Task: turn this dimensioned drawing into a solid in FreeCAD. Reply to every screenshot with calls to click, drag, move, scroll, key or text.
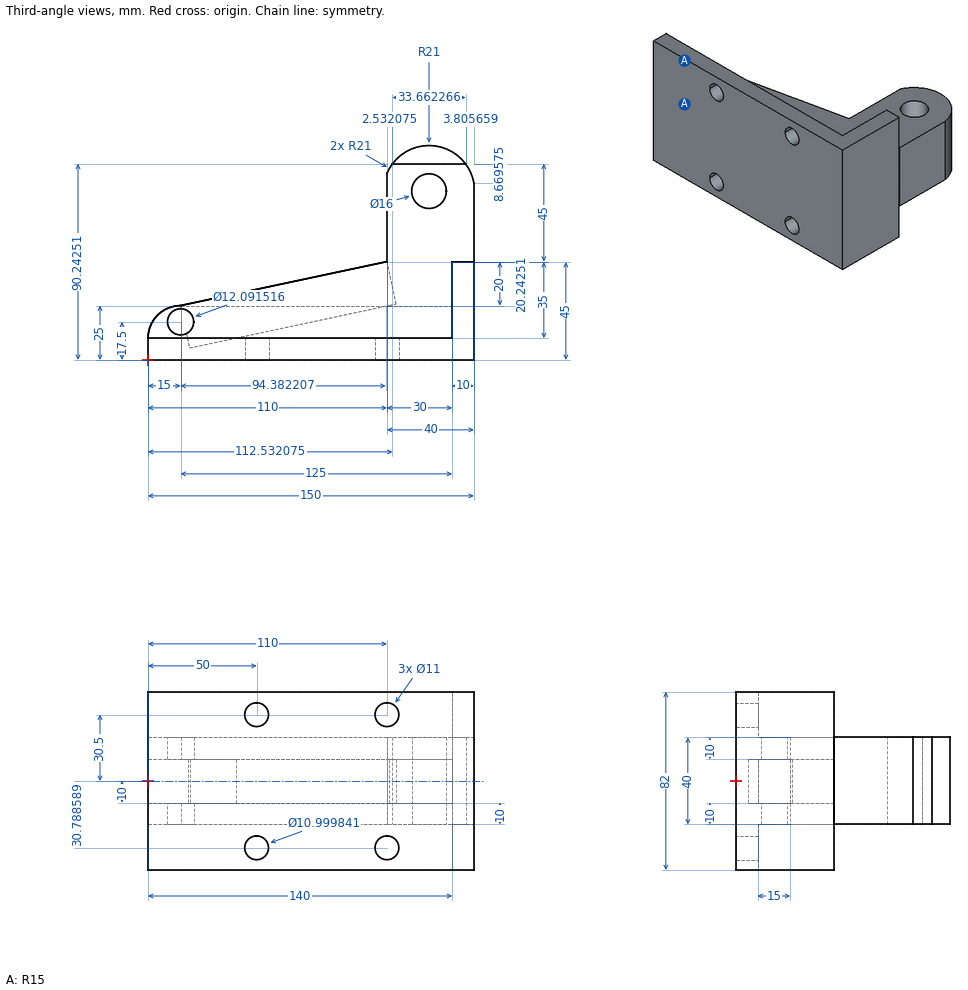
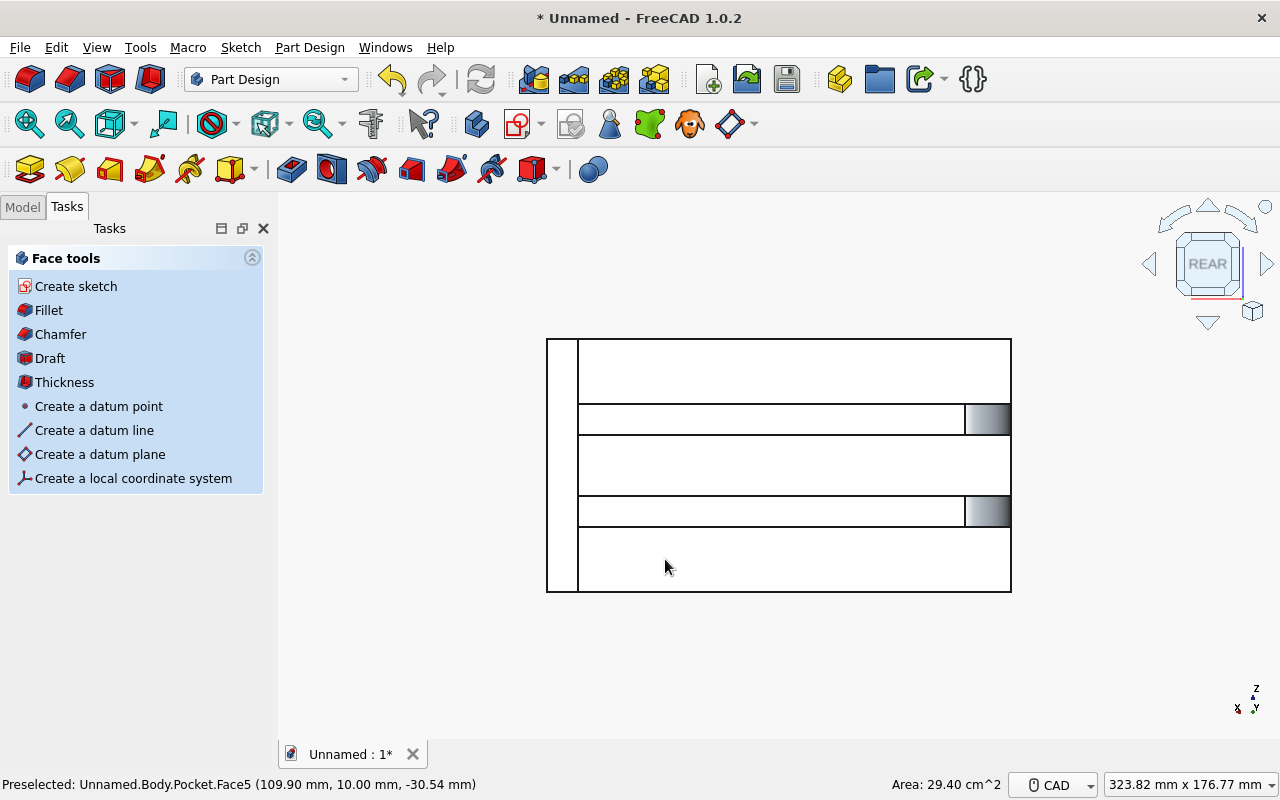
click(518, 124)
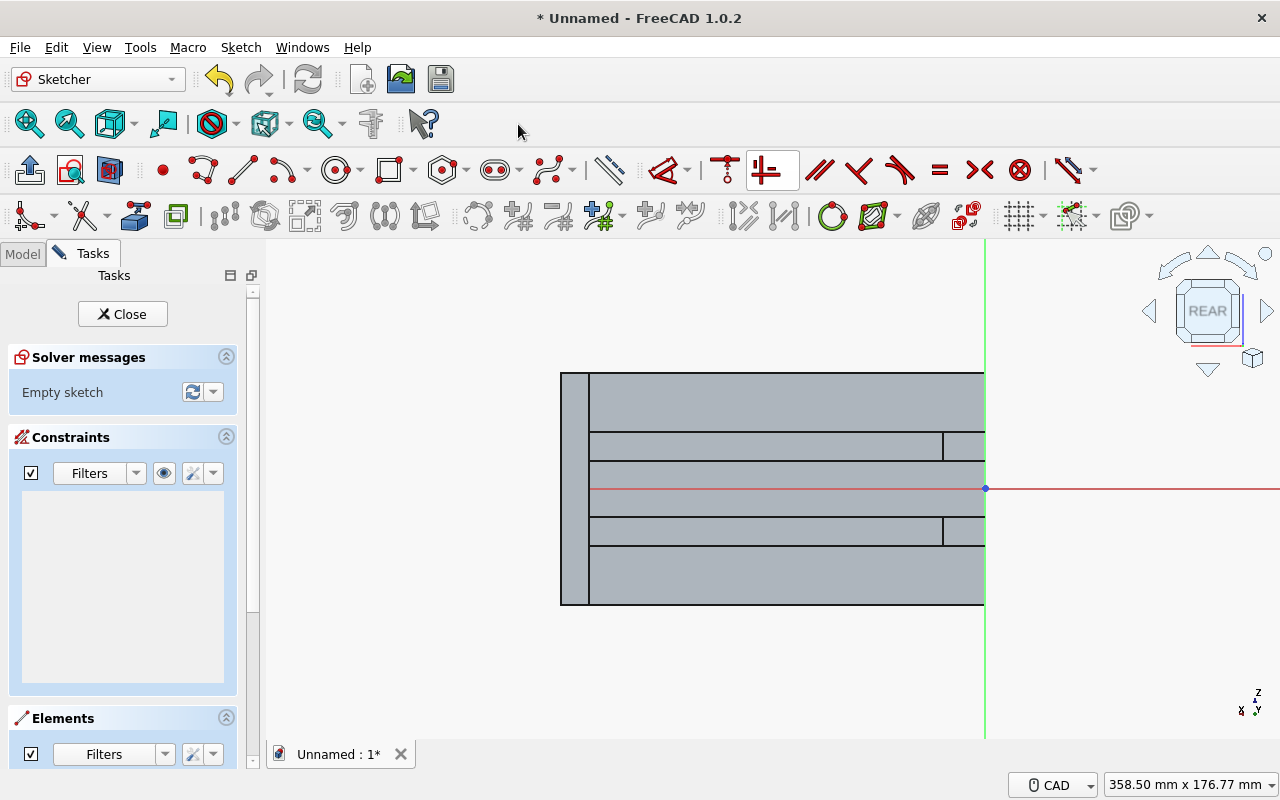
click(110, 170)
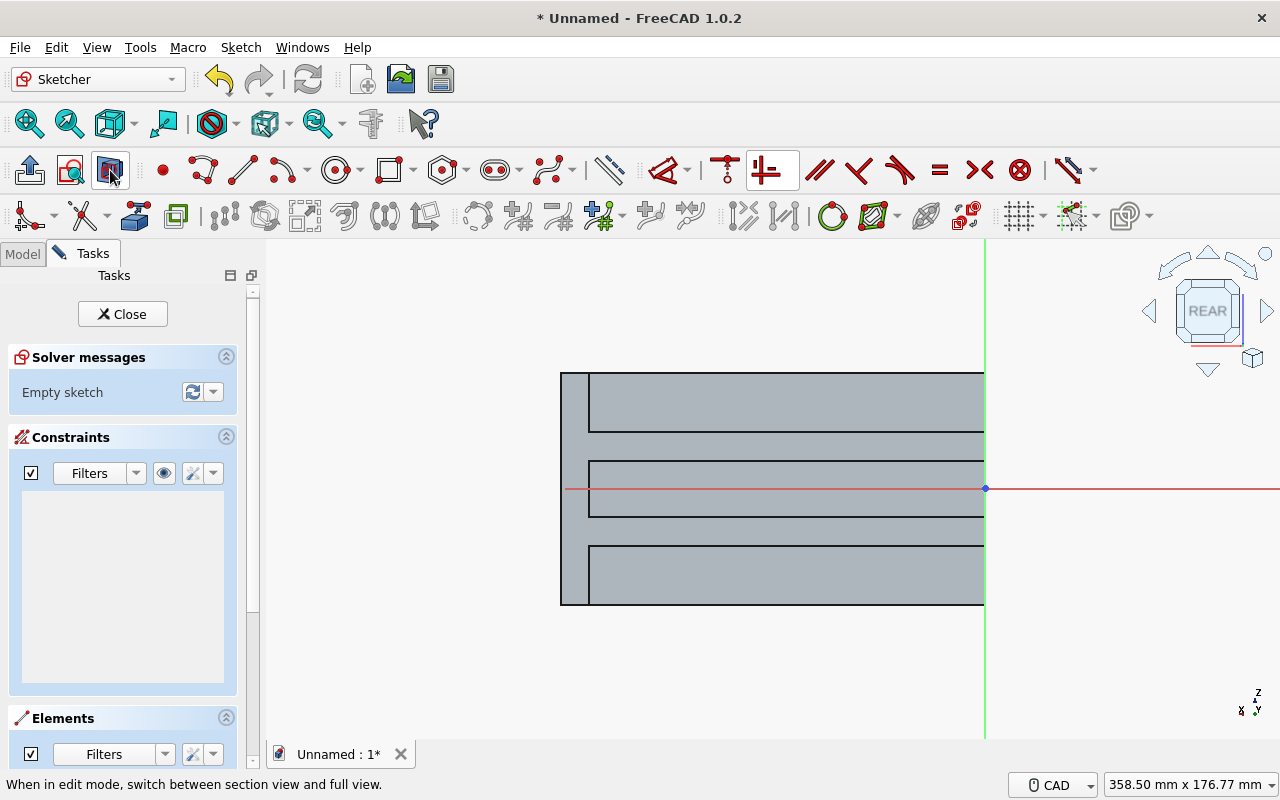
scroll(1060, 490, up, 2)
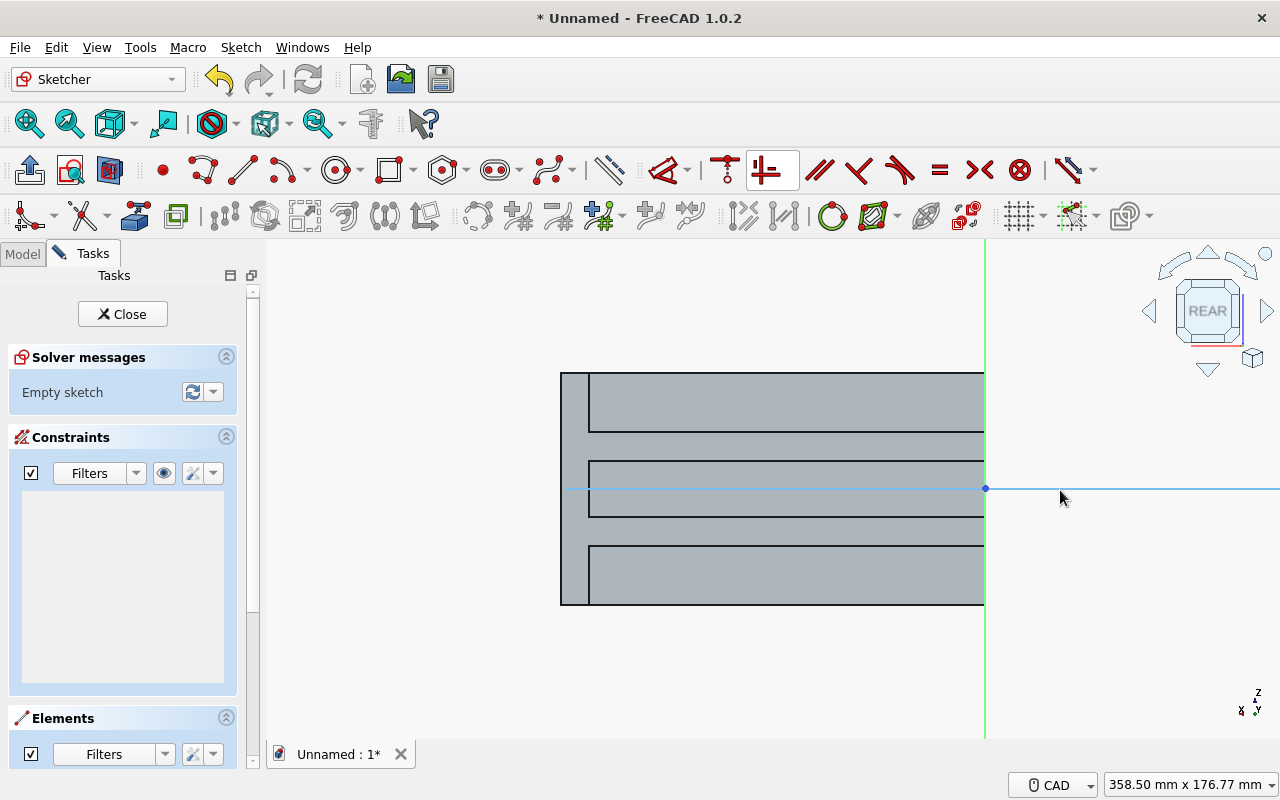
click(336, 170)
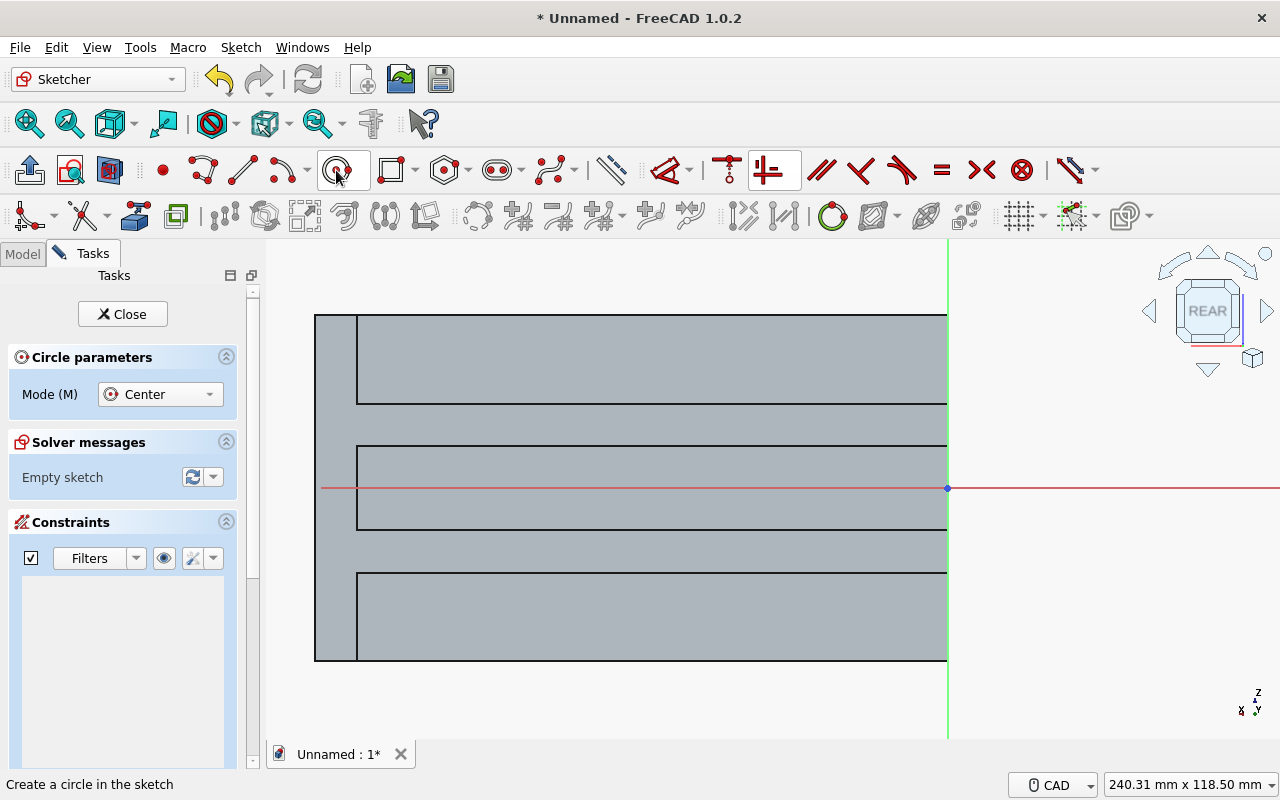
click(484, 360)
move(500, 343)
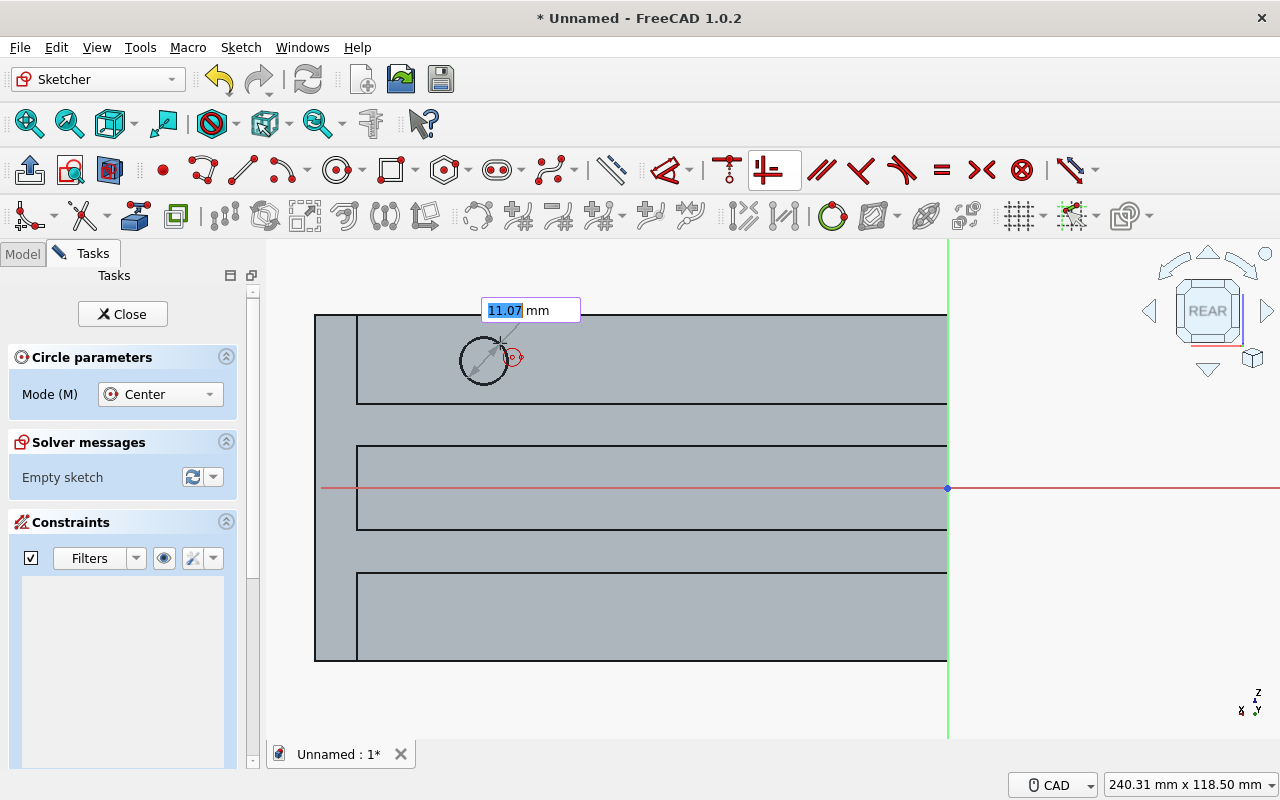
text(11)
key(Return)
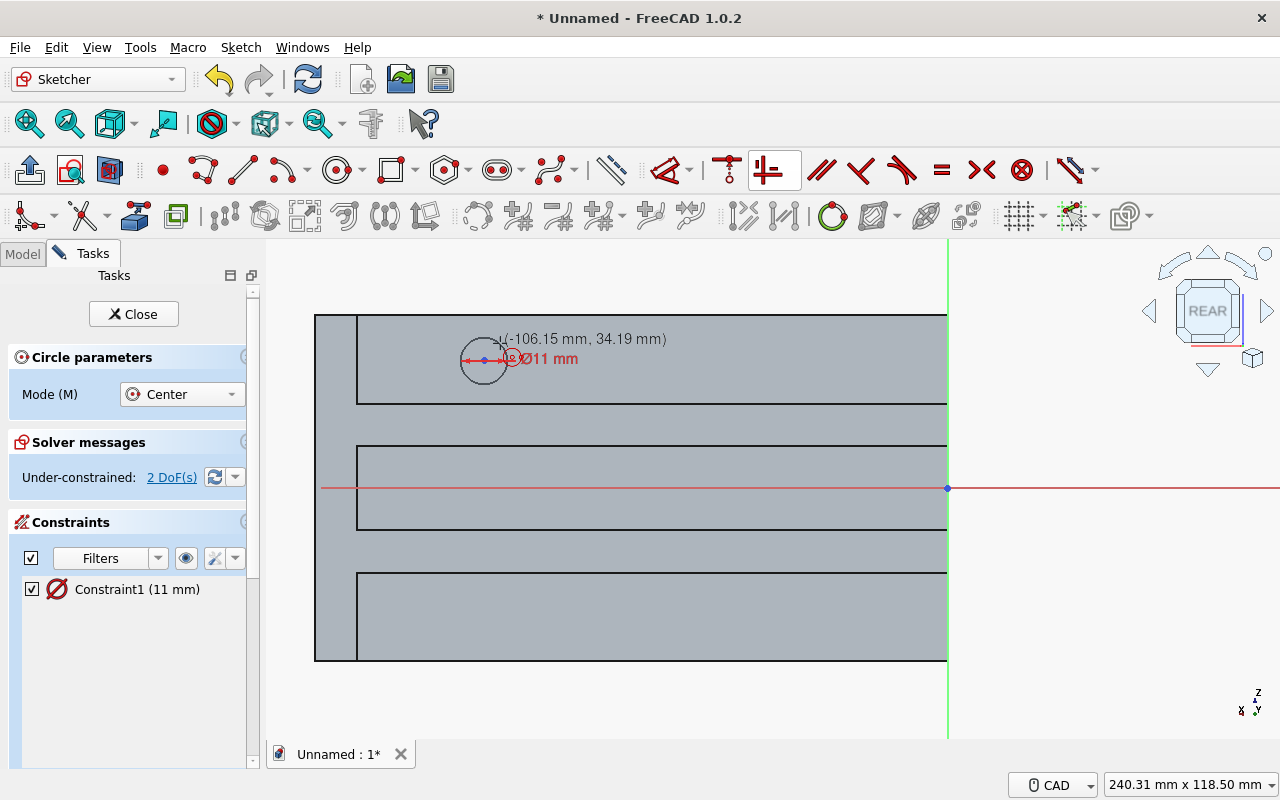
click(737, 360)
move(753, 343)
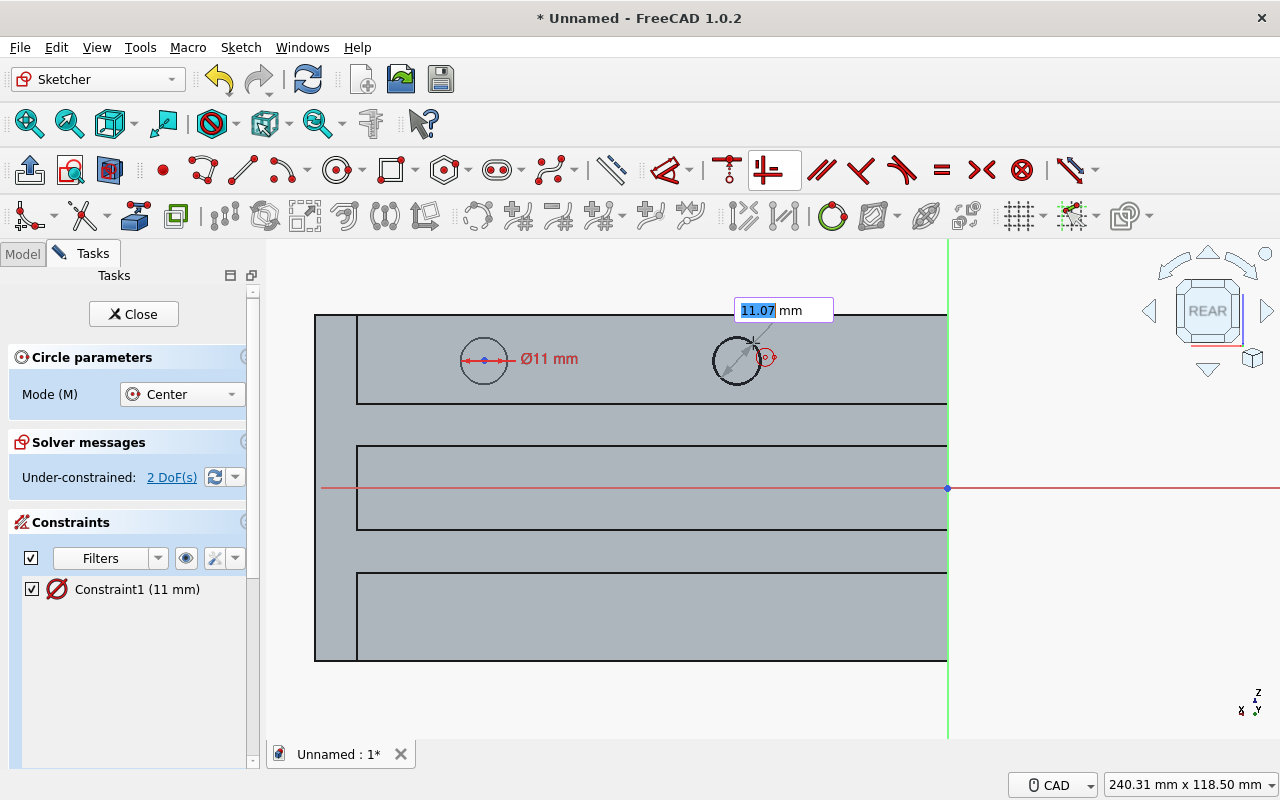
text(11)
key(Return)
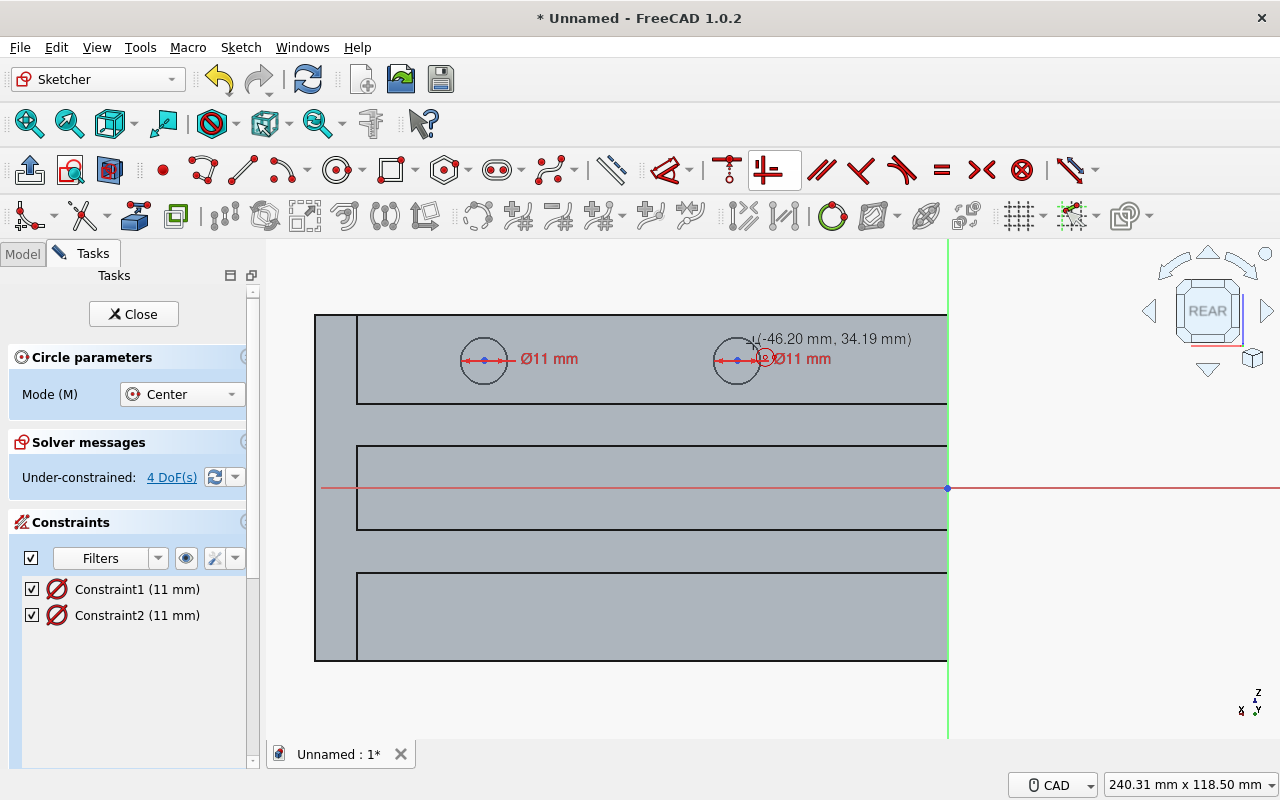
click(484, 618)
move(500, 602)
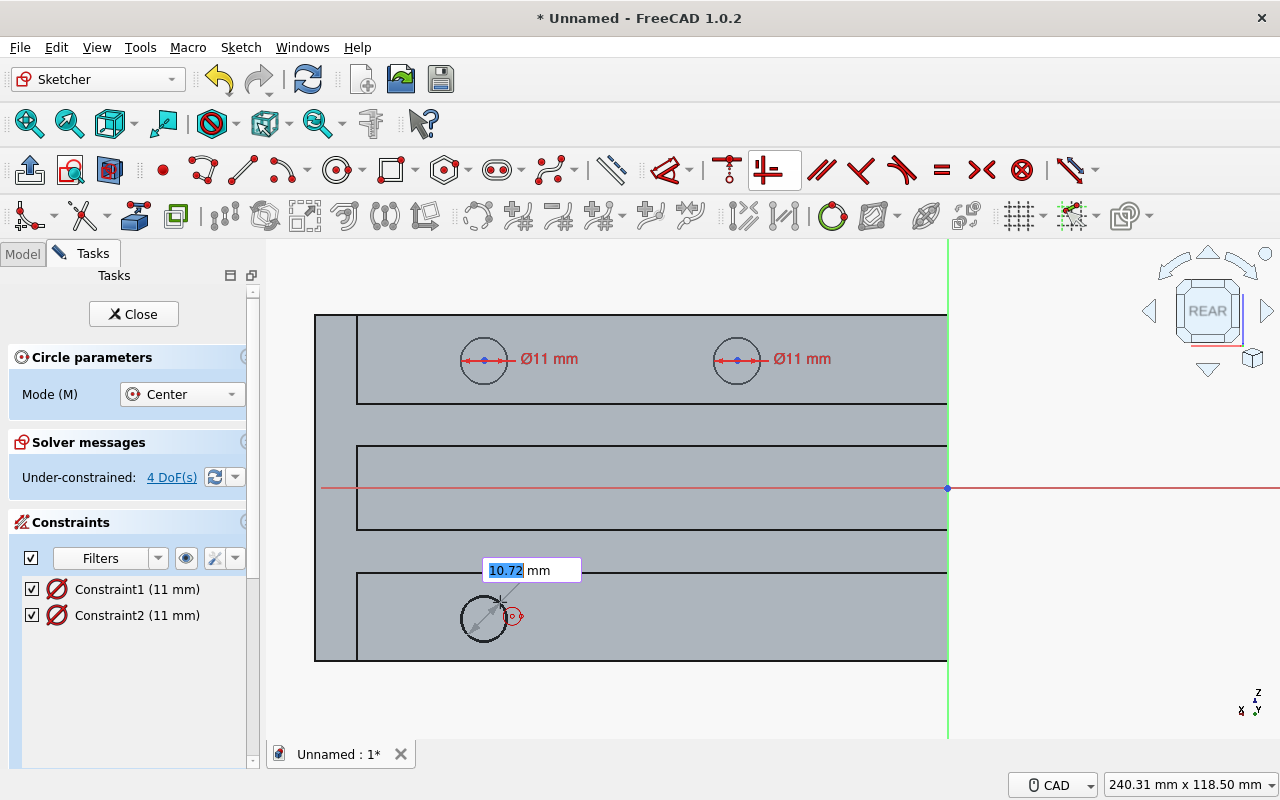
text(11)
key(Return)